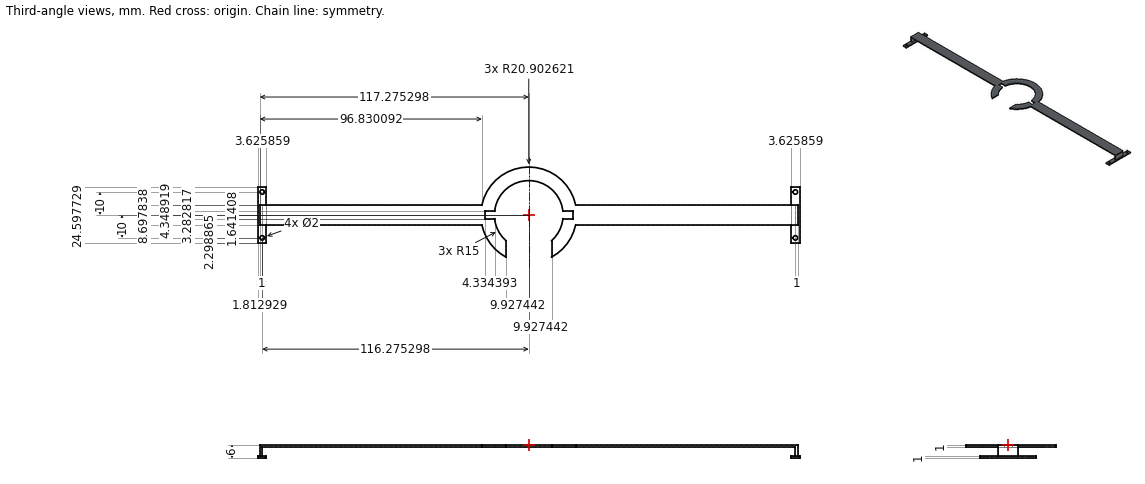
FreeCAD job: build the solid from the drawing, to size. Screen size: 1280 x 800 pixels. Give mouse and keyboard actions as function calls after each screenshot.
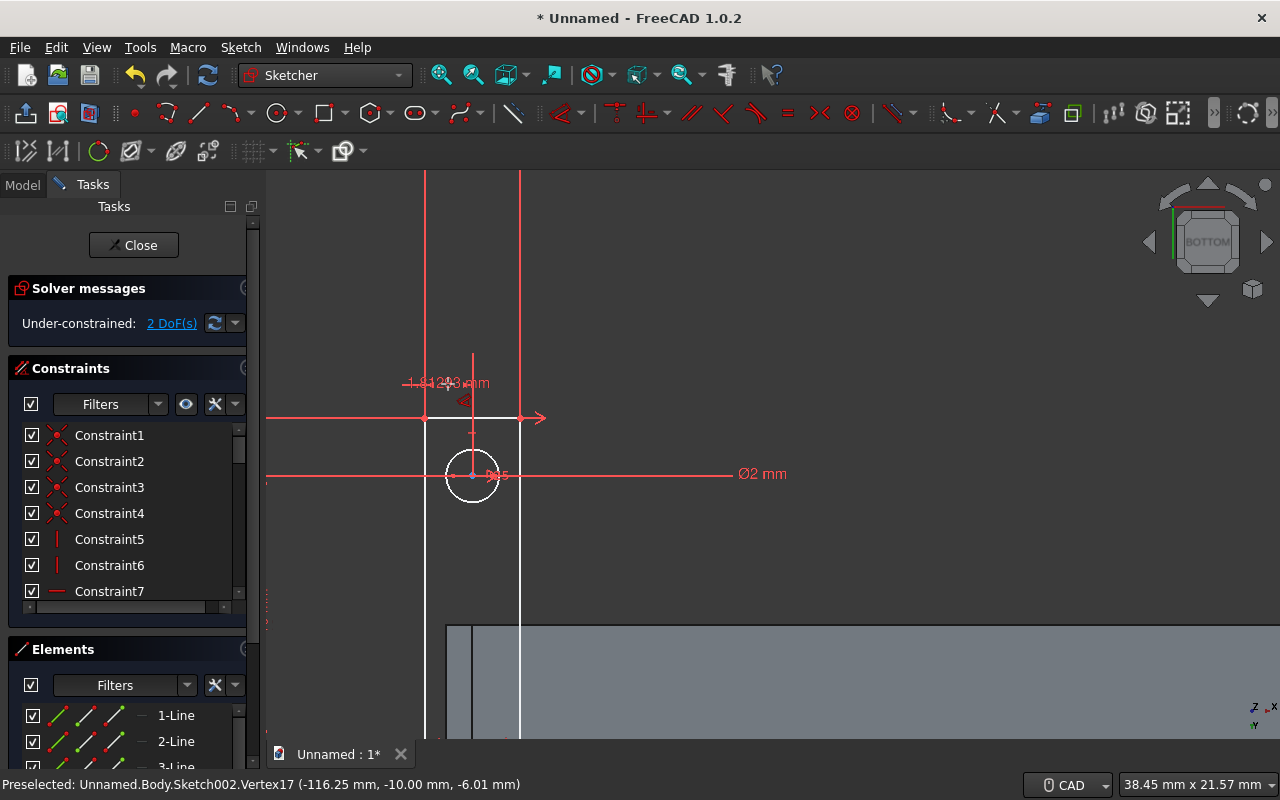
click(425, 418)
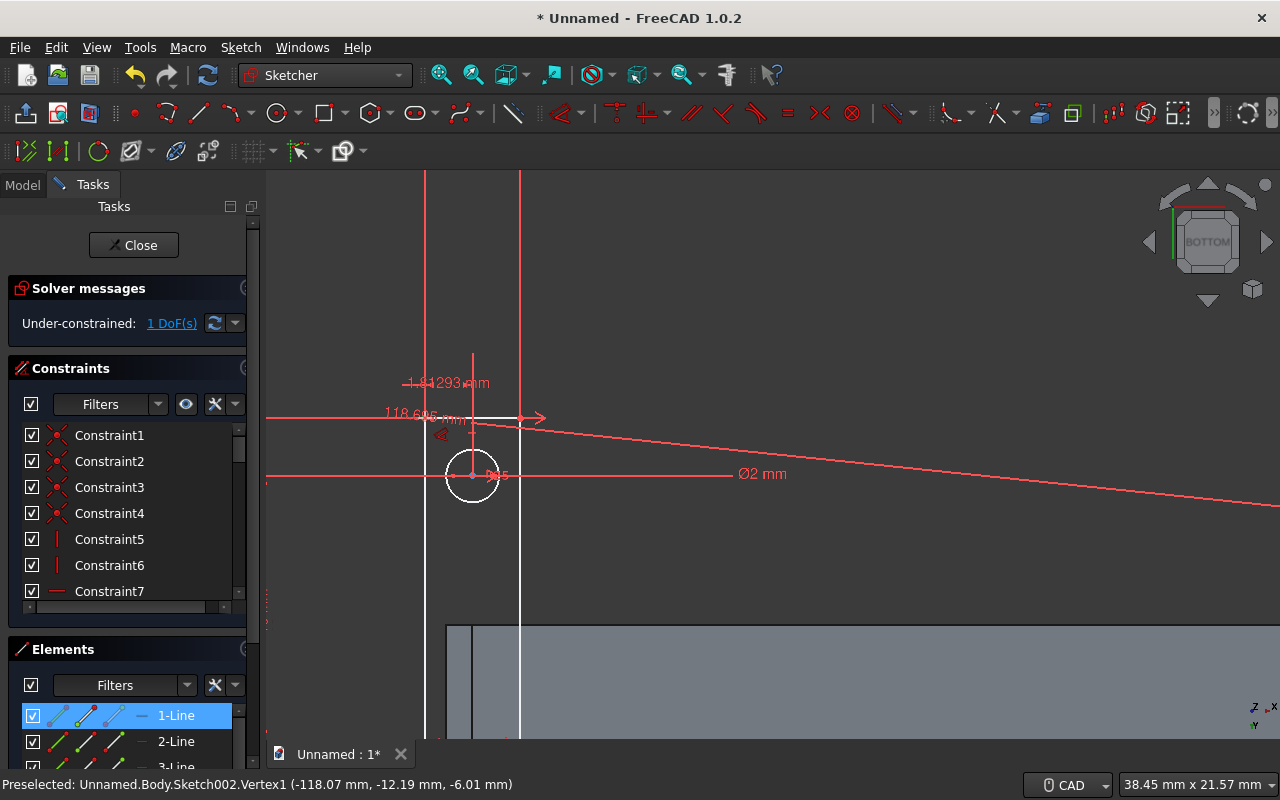
click(473, 476)
click(391, 447)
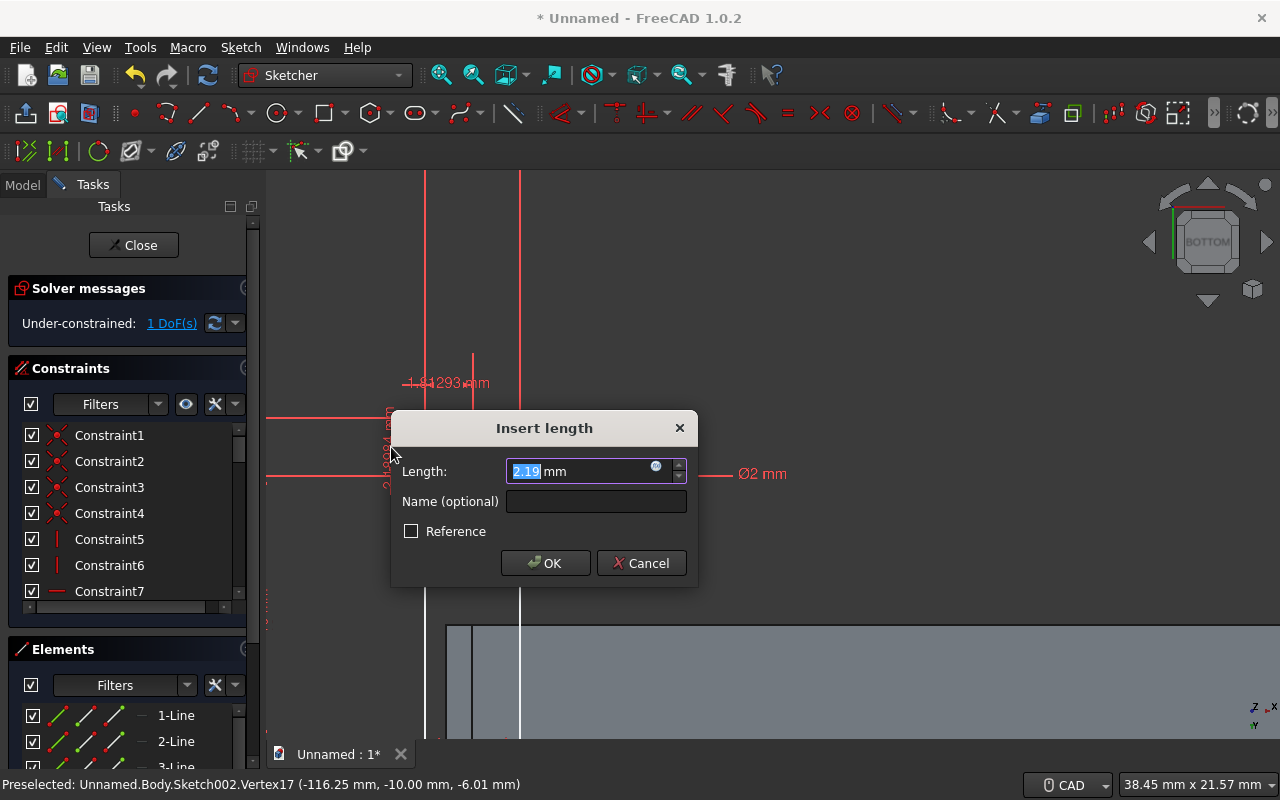
text(2.298865)
key(Return)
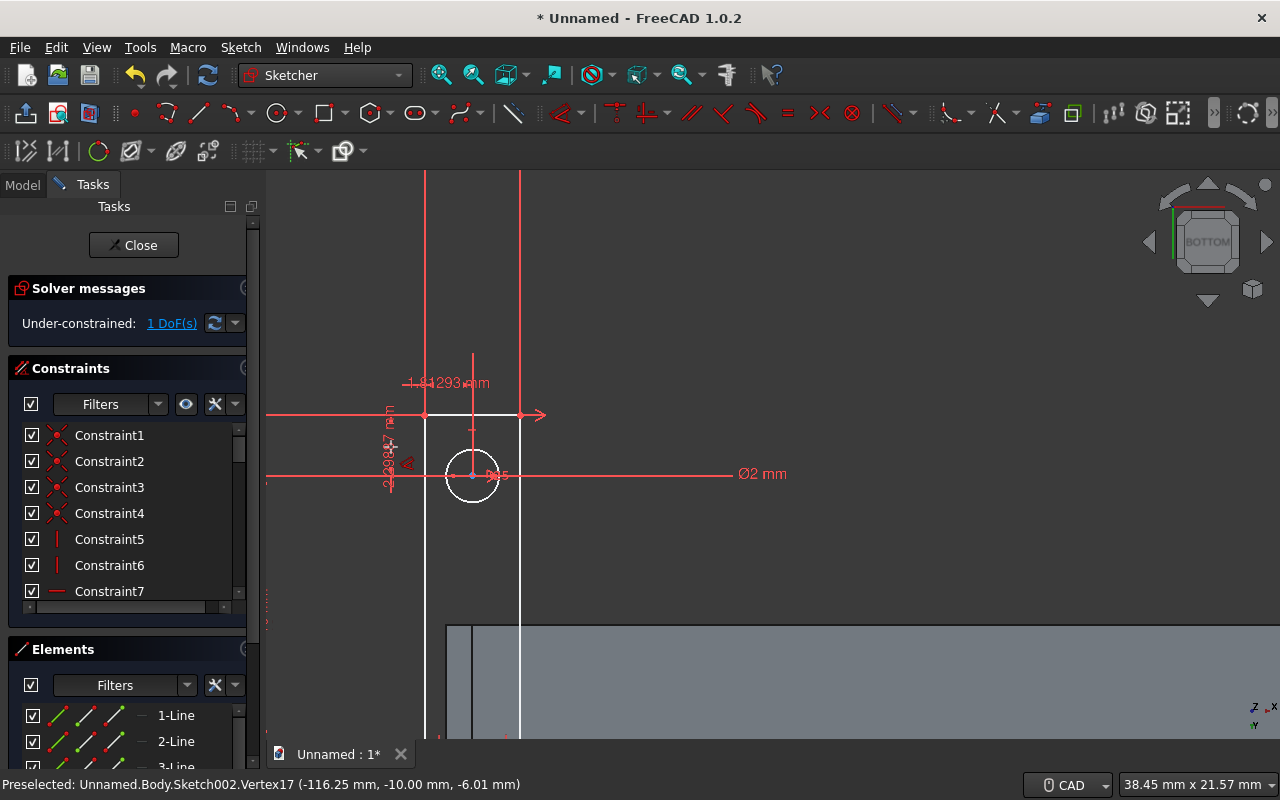
scroll(422, 426, down, 12)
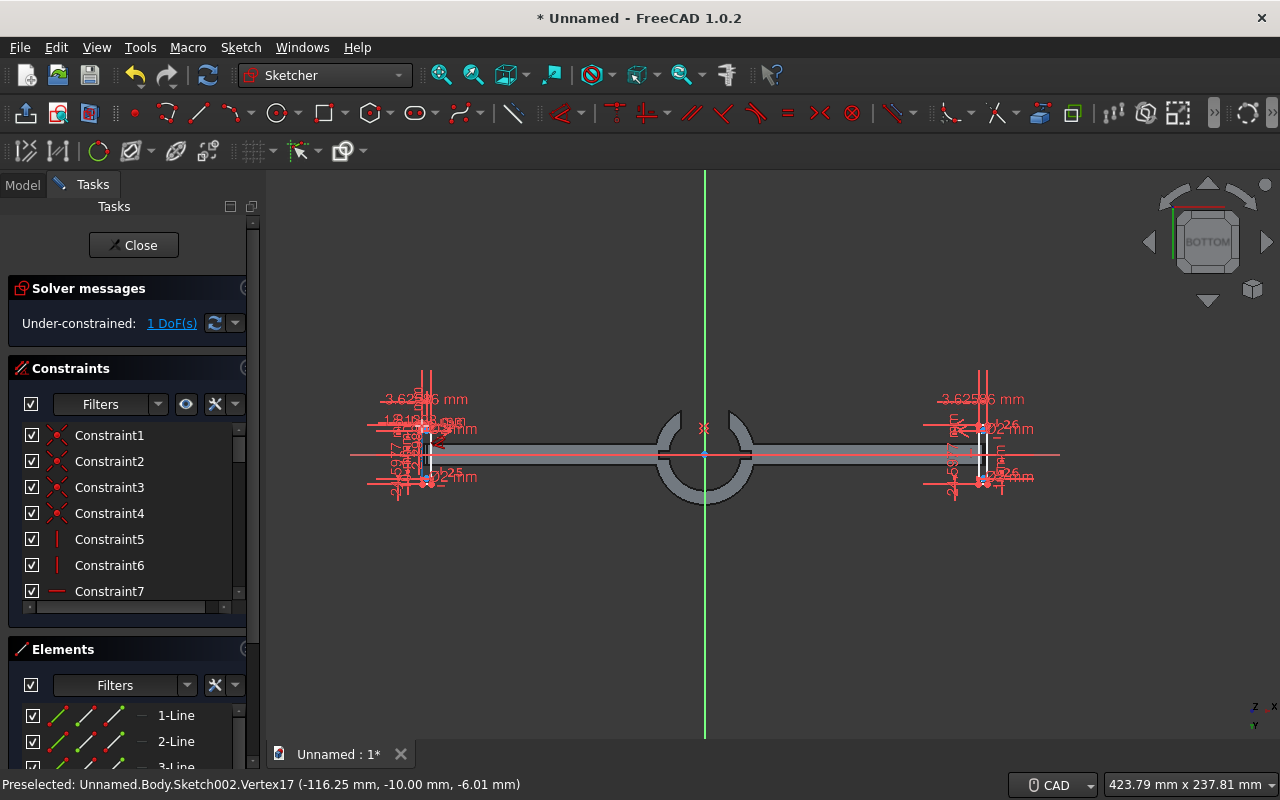
scroll(427, 431, up, 3)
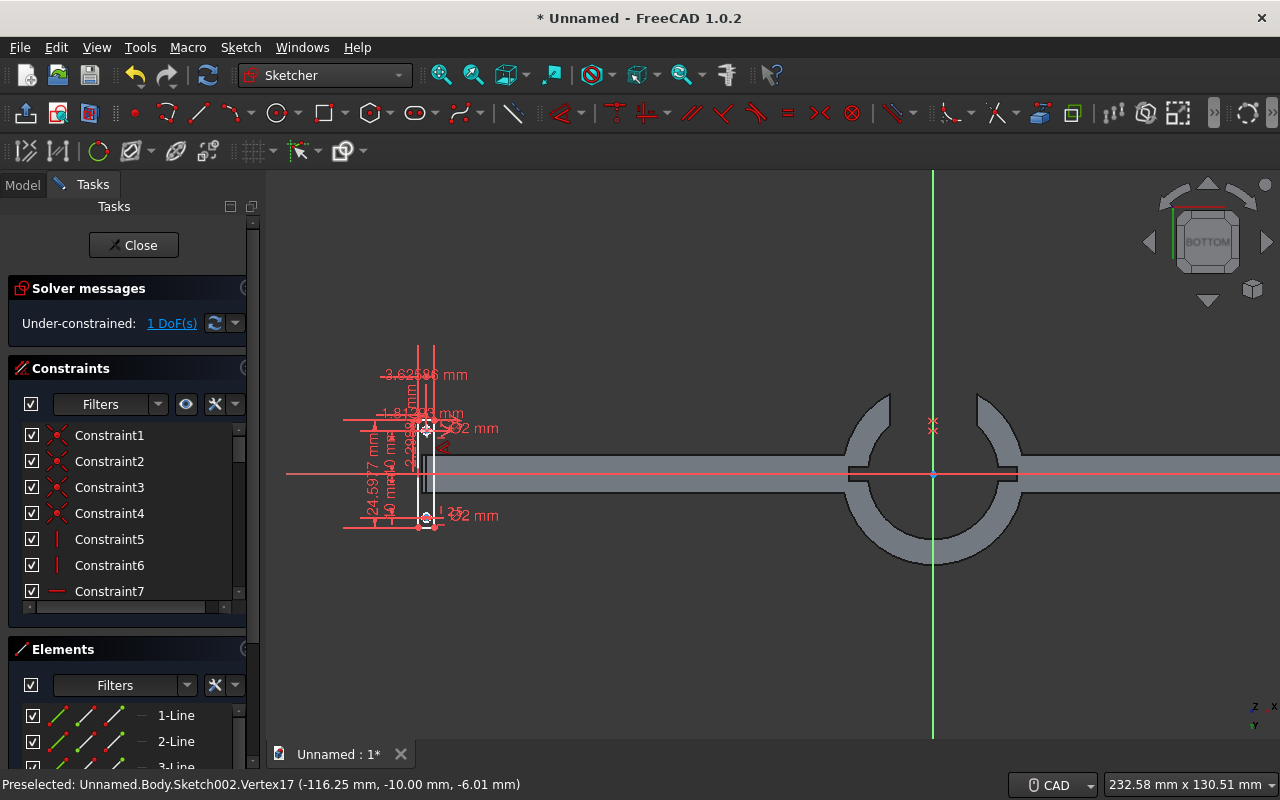
click(426, 431)
click(680, 397)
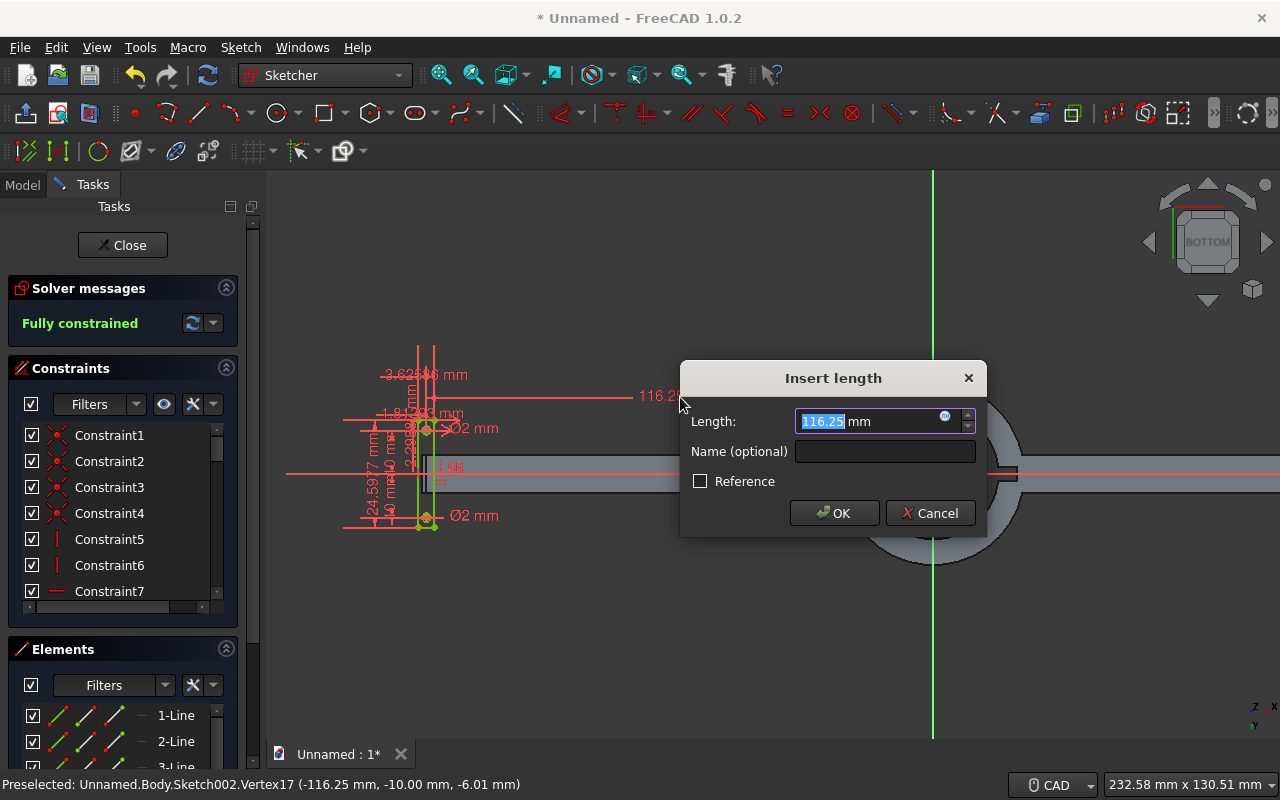
text(116.275298)
key(Return)
key(Escape)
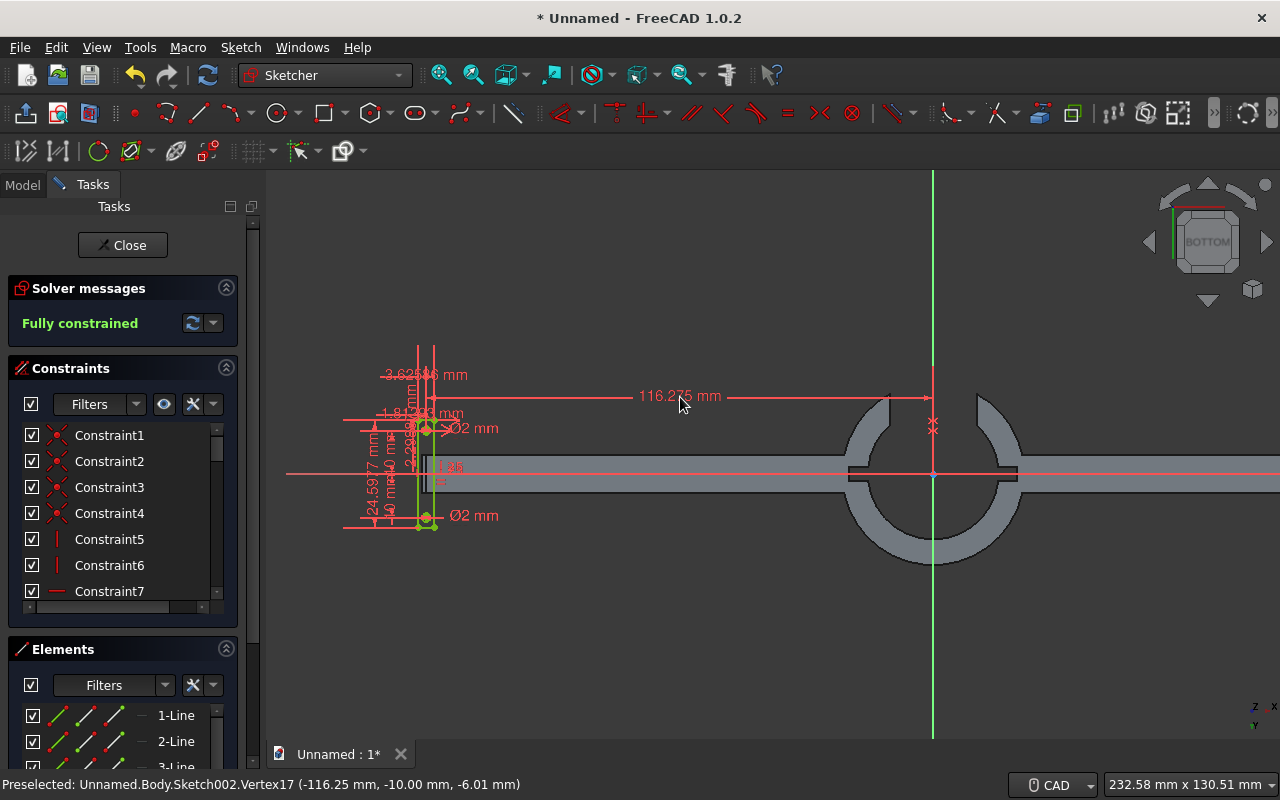
click(123, 245)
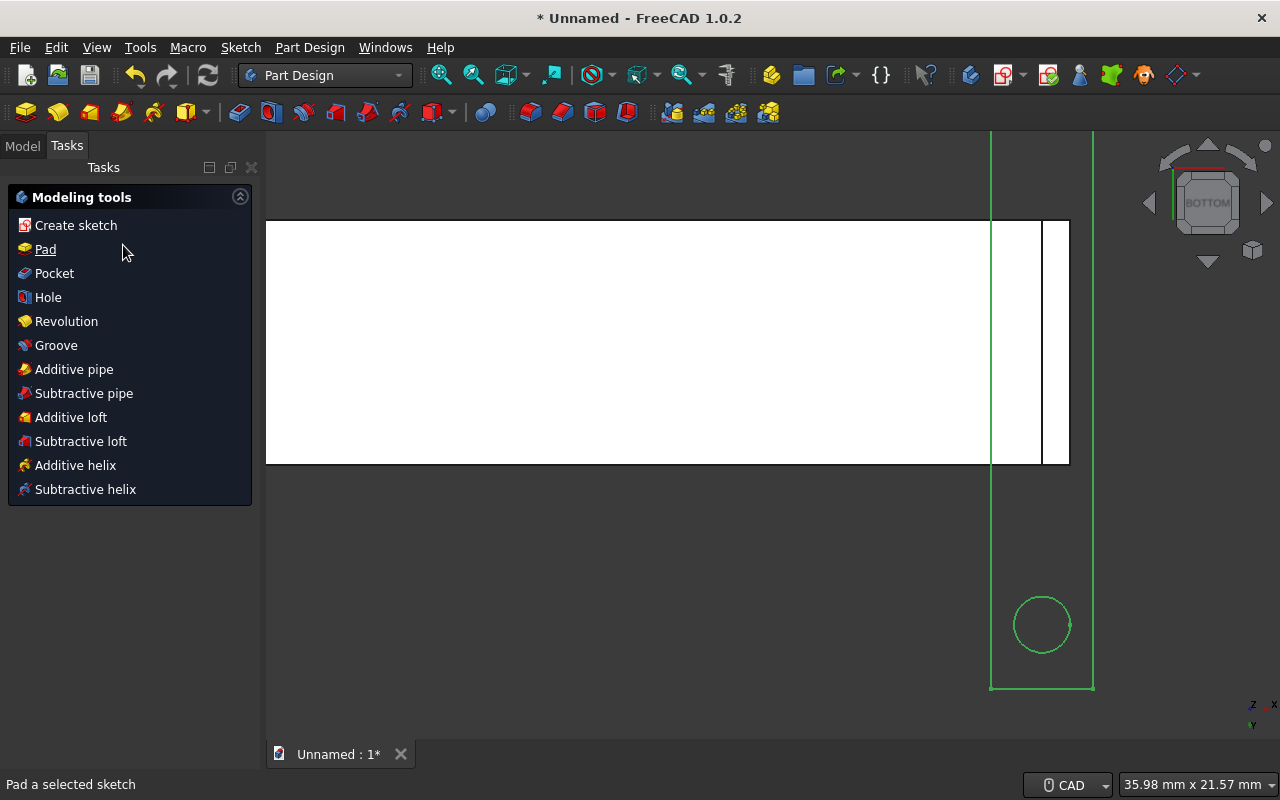
click(26, 112)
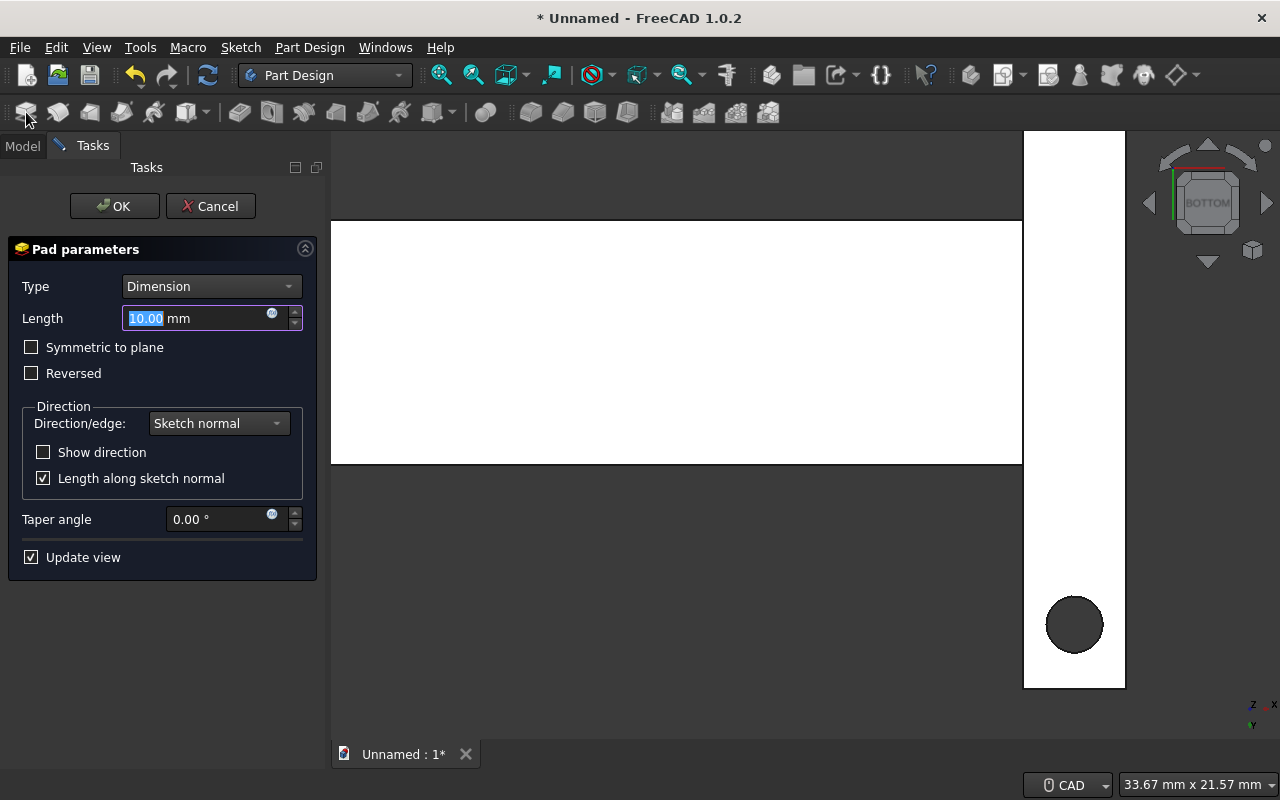
text(1)
key(Tab)